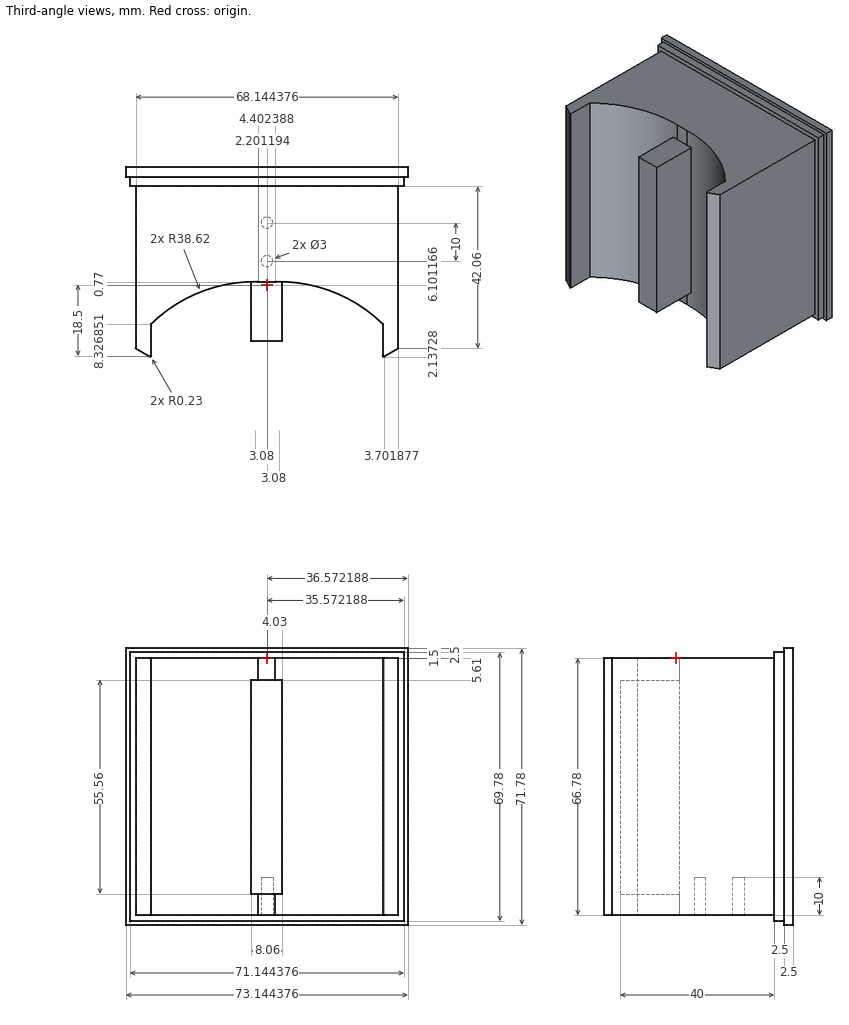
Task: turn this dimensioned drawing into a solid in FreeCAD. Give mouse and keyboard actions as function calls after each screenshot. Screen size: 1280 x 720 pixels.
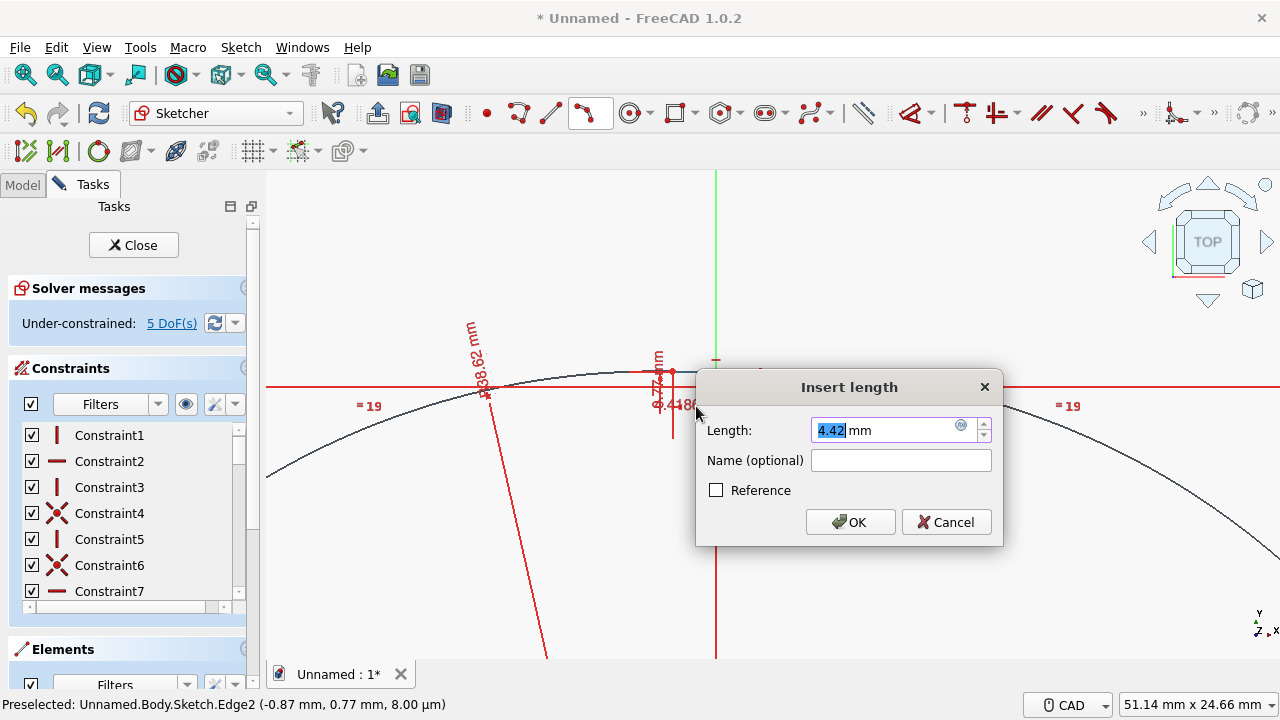
text(4.402388)
key(Return)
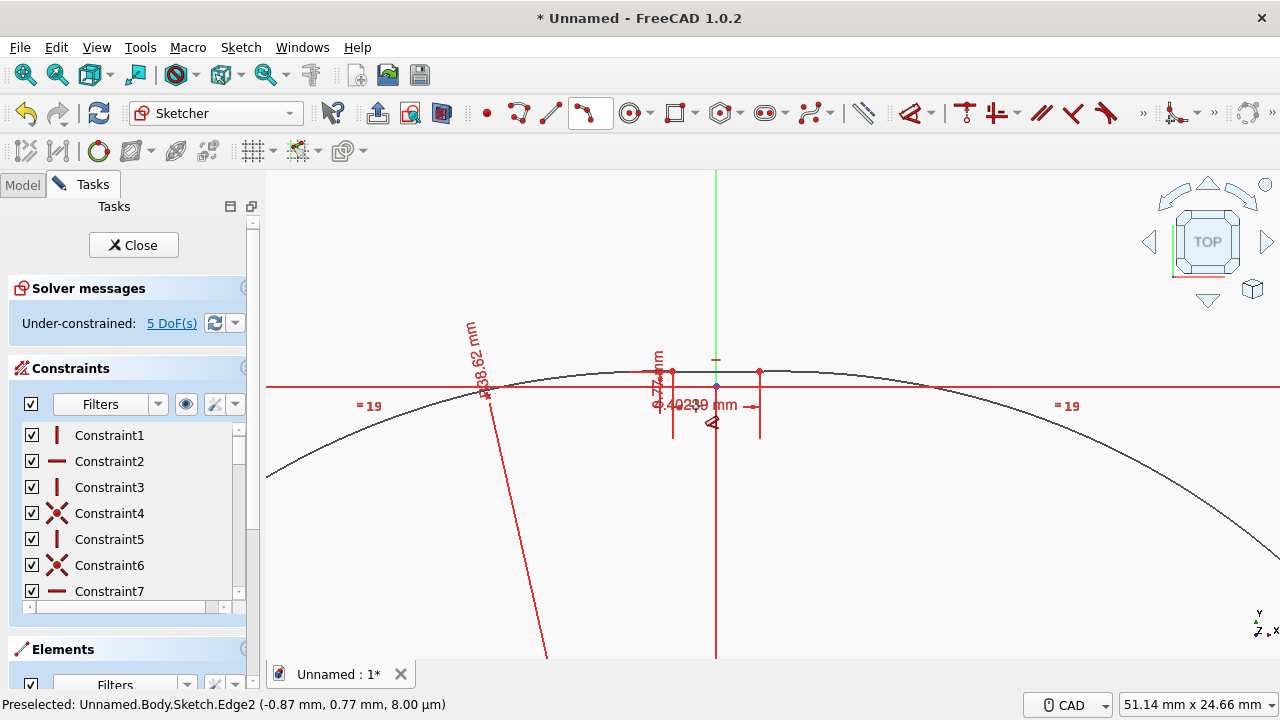
scroll(698, 470, down, 5)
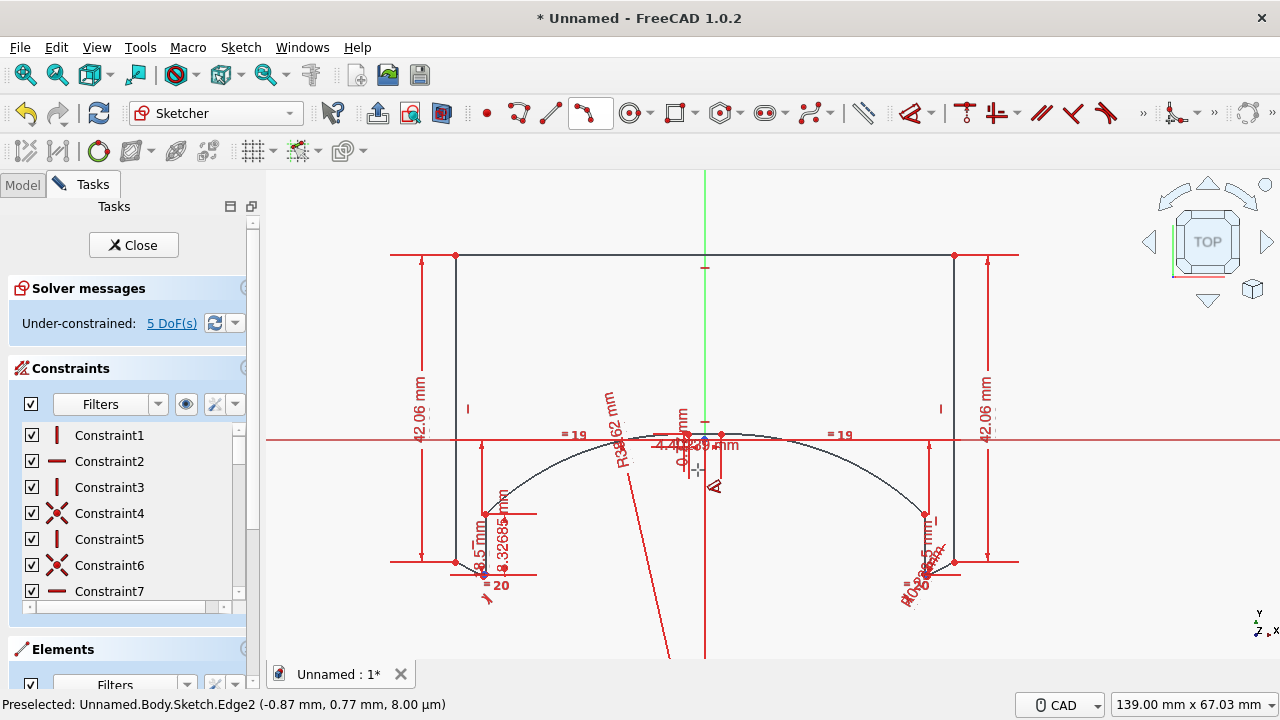
click(925, 533)
click(891, 524)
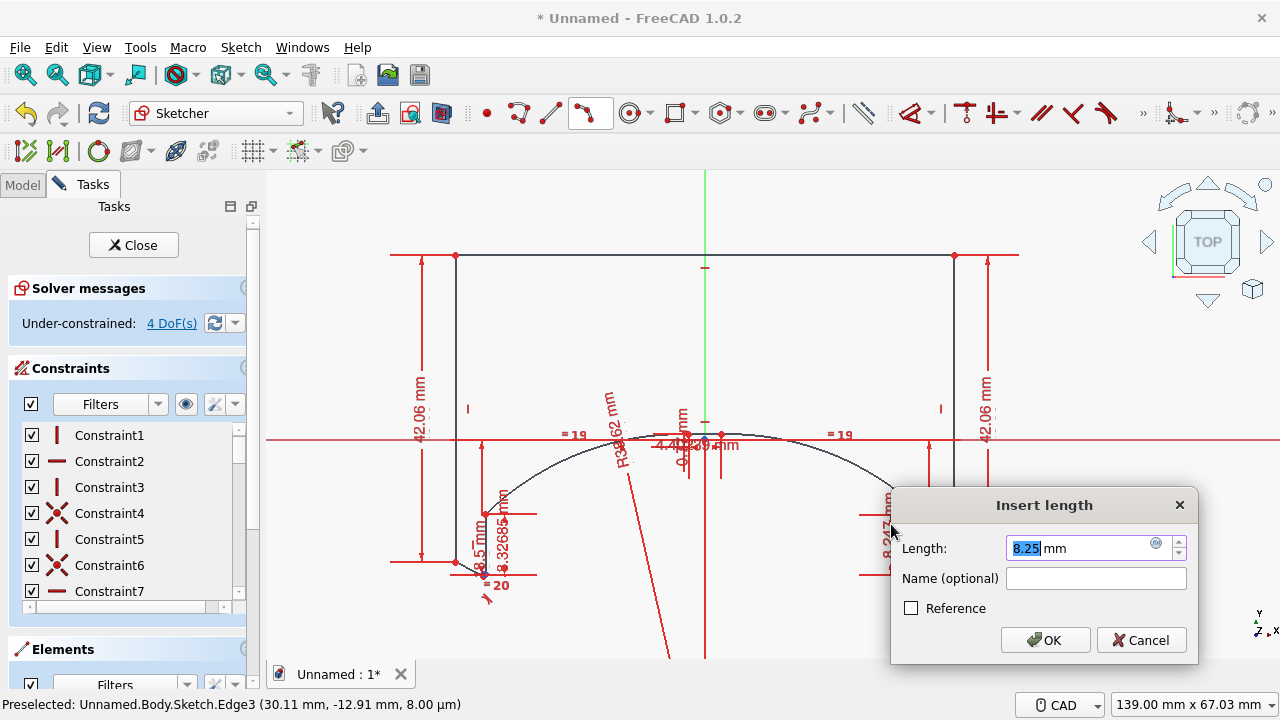
text(8.326851)
key(Return)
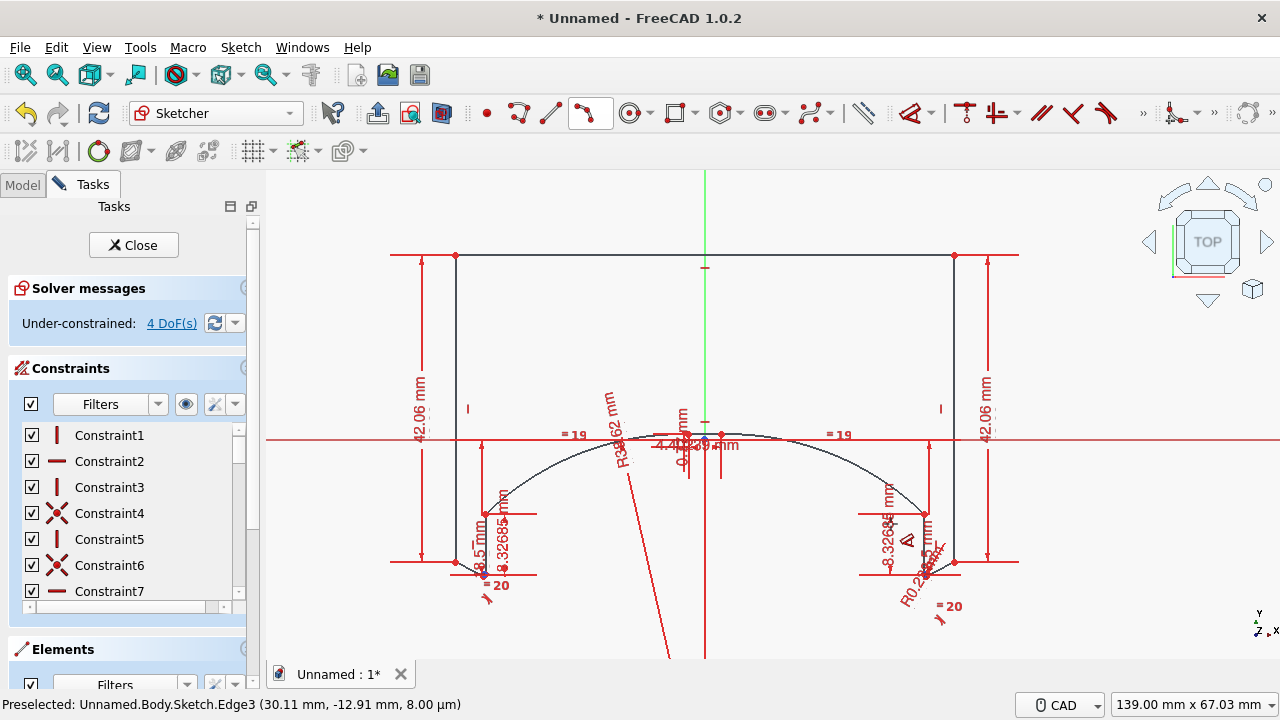
scroll(935, 572, up, 5)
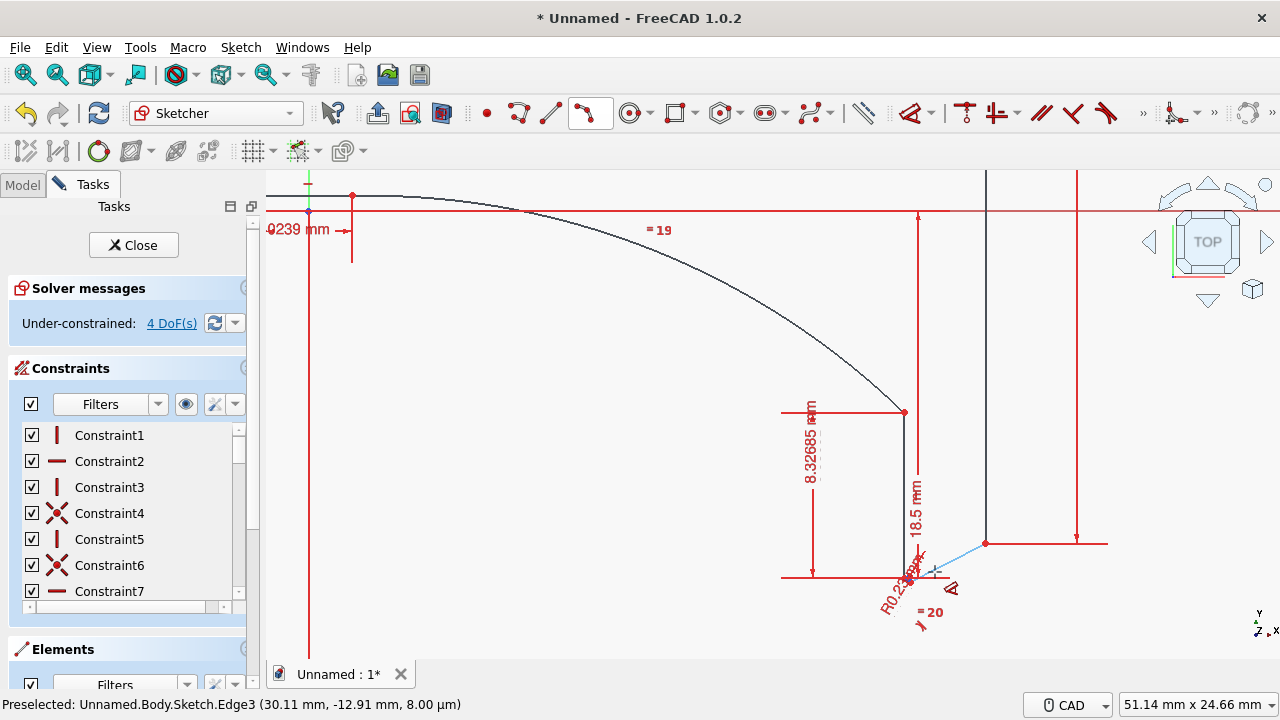
click(933, 571)
click(1020, 563)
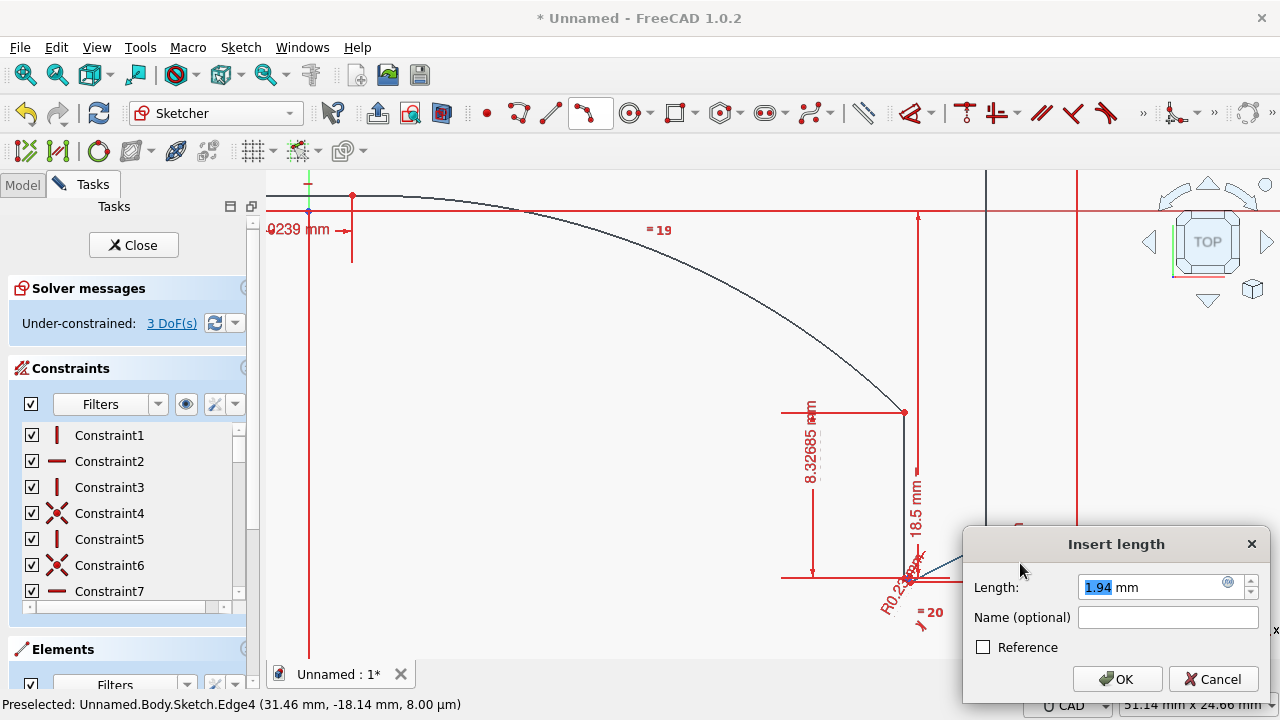
text(2.13728)
key(Return)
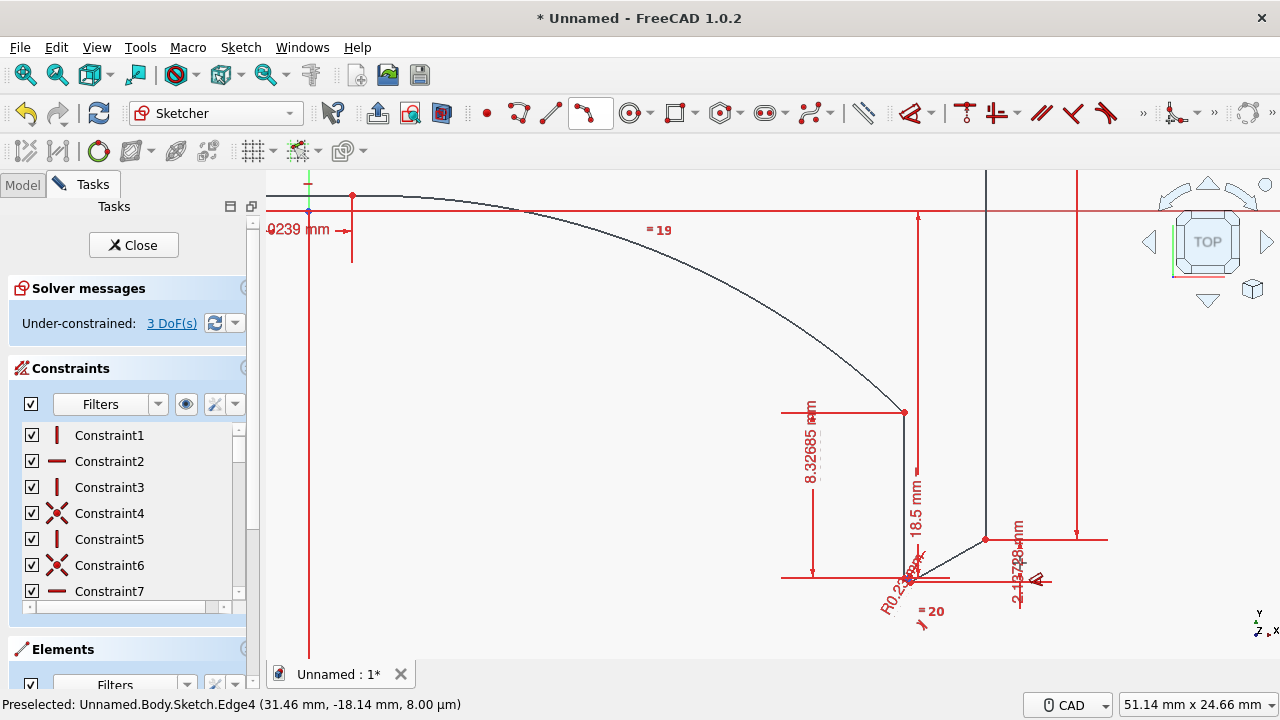
scroll(935, 572, down, 5)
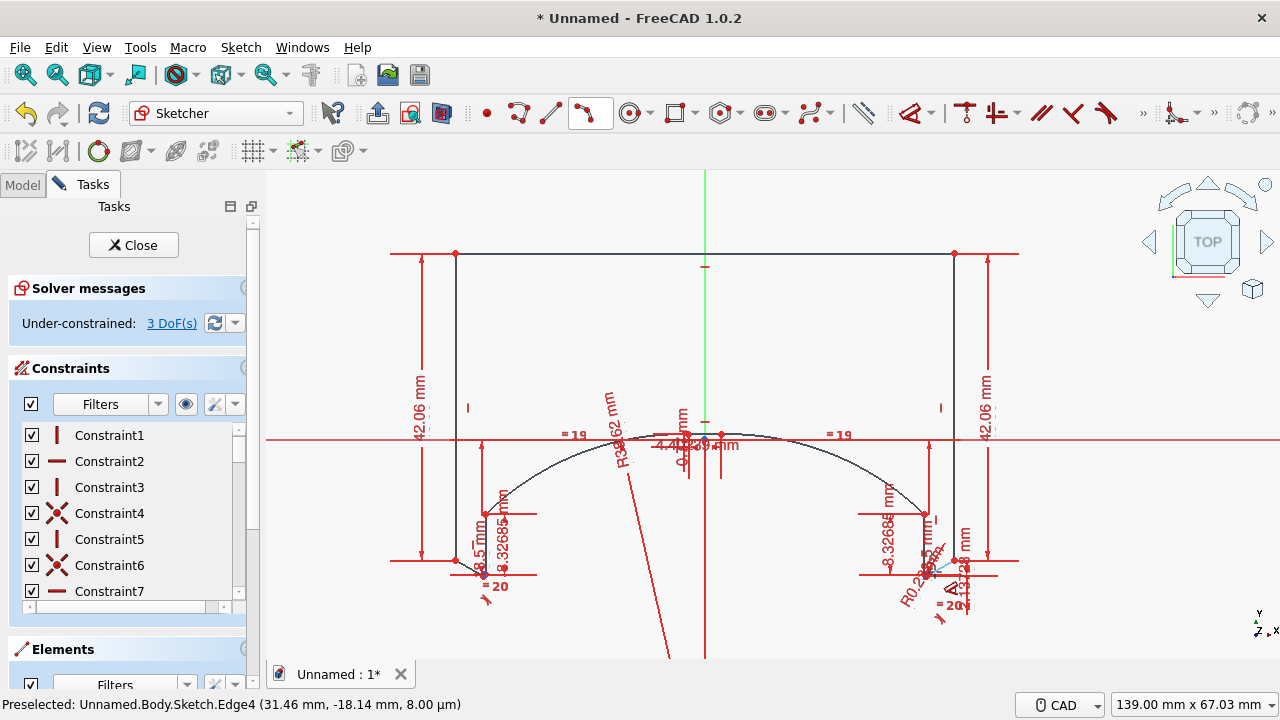
click(805, 254)
click(590, 220)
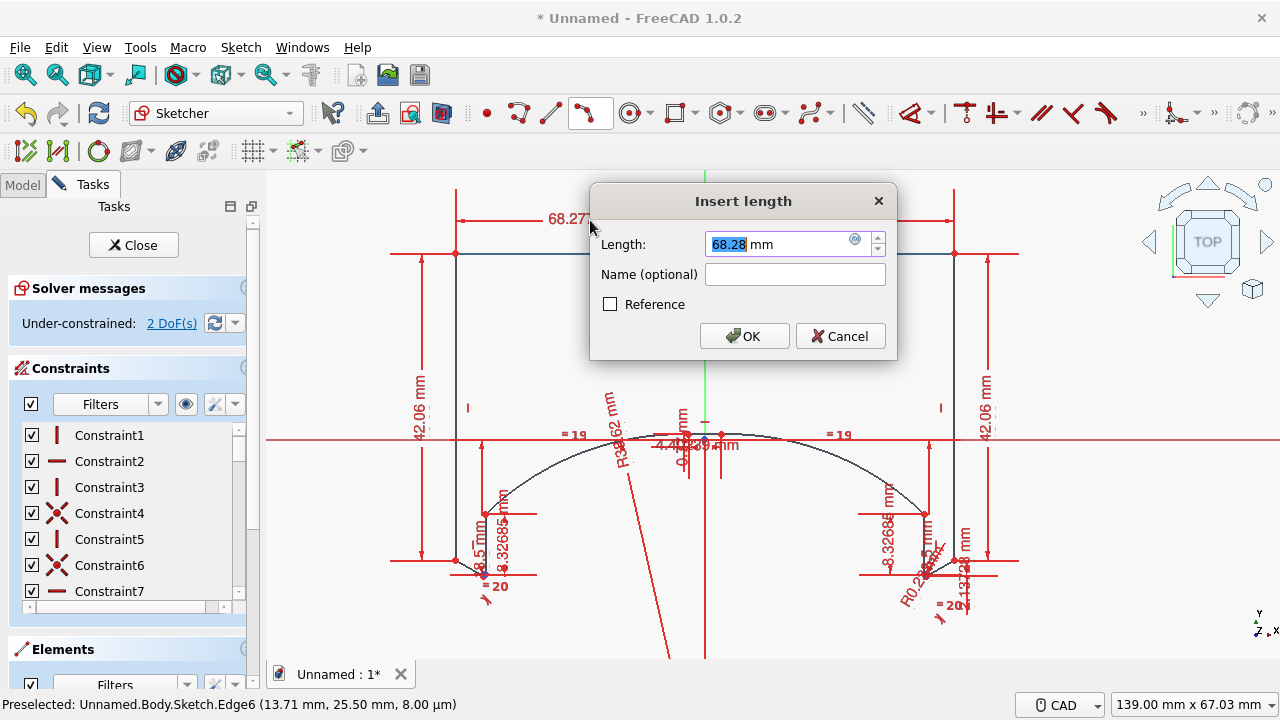
text(68.144376)
key(Return)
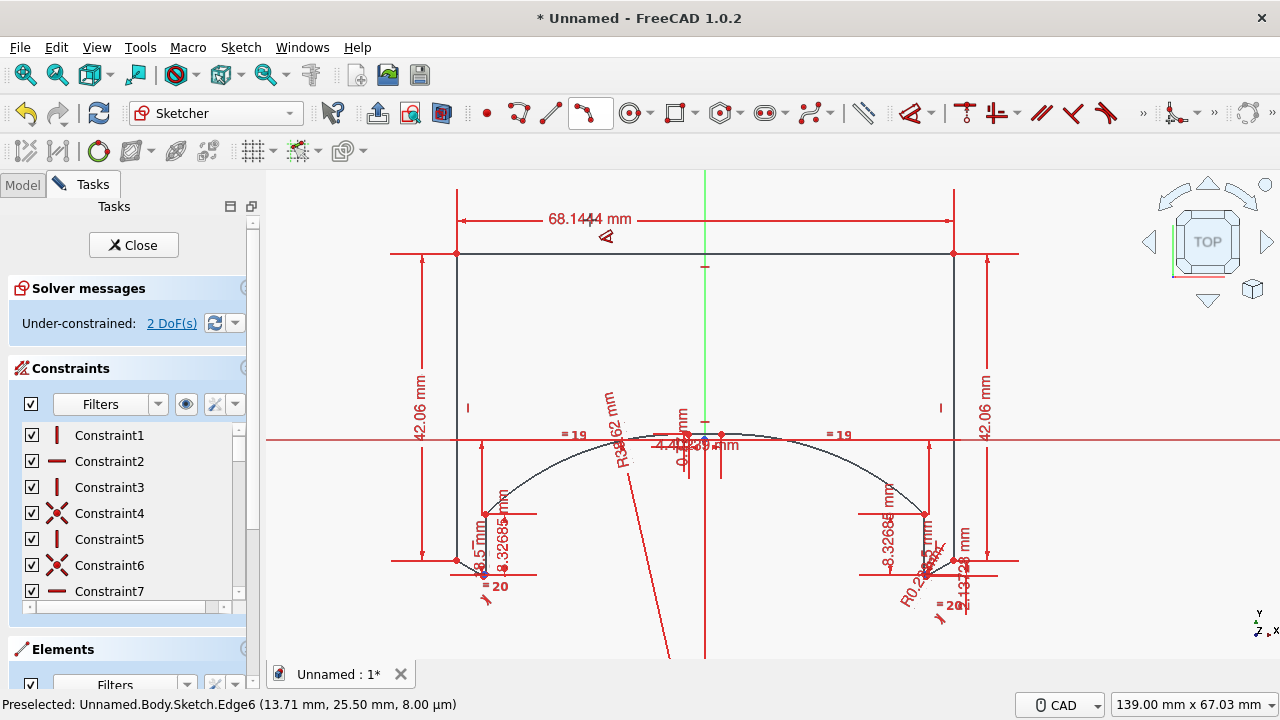
scroll(689, 434, up, 5)